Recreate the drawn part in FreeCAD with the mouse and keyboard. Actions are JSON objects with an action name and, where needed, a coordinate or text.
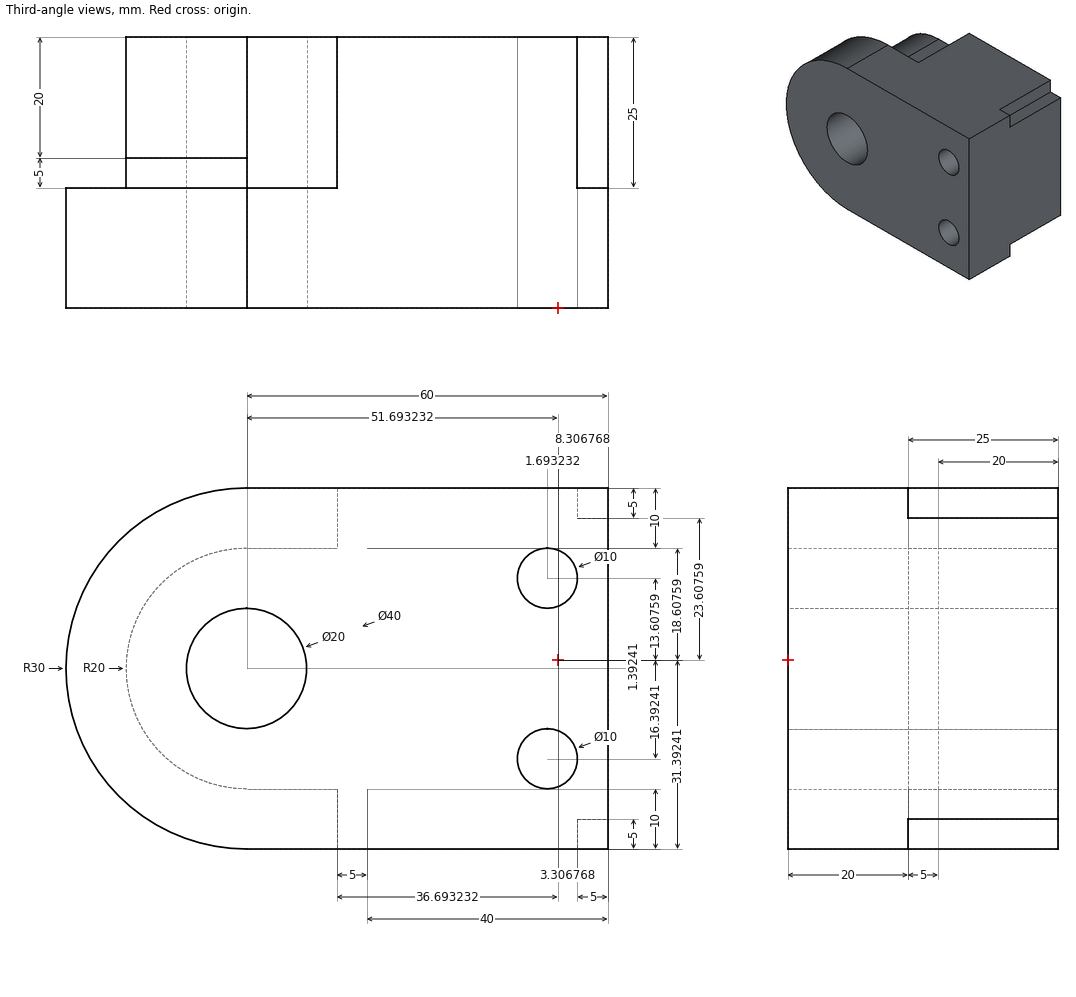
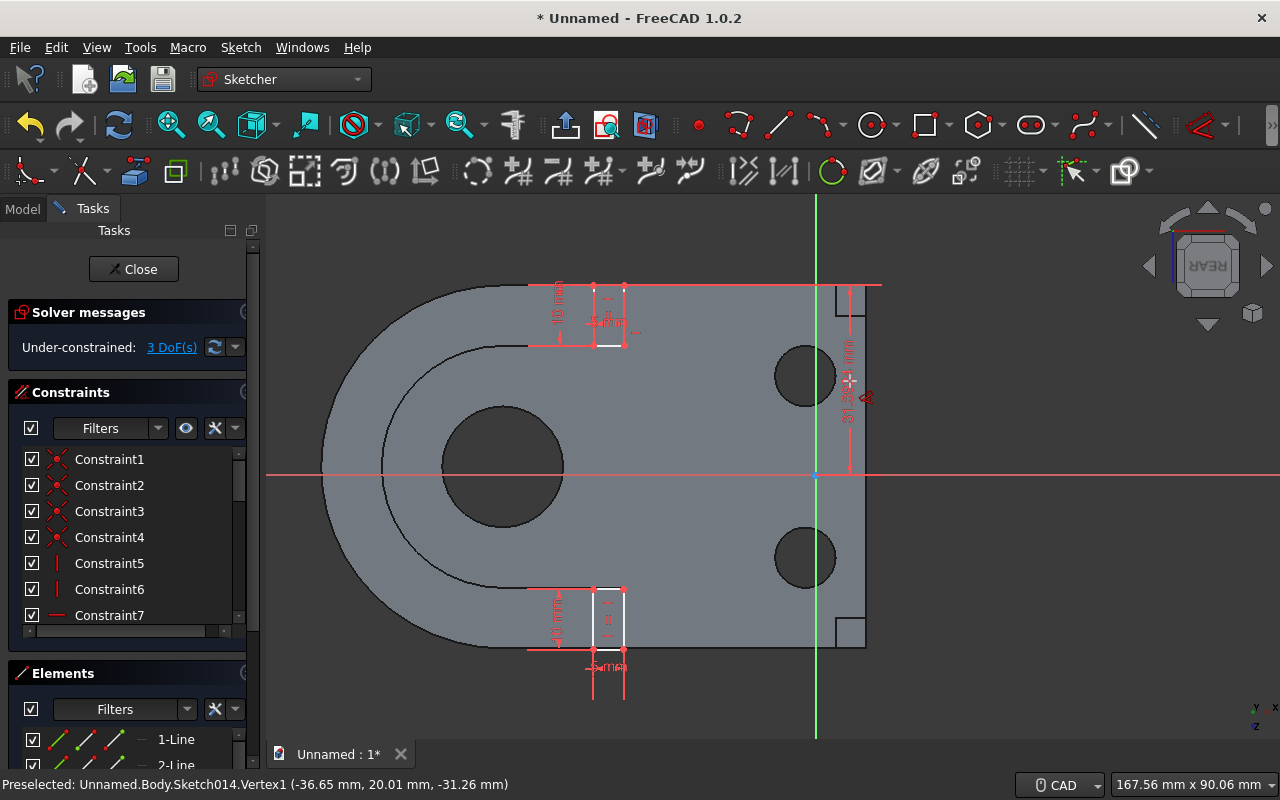
{"action": "left_click", "coordinate": [593, 589]}
{"action": "left_click", "coordinate": [850, 532]}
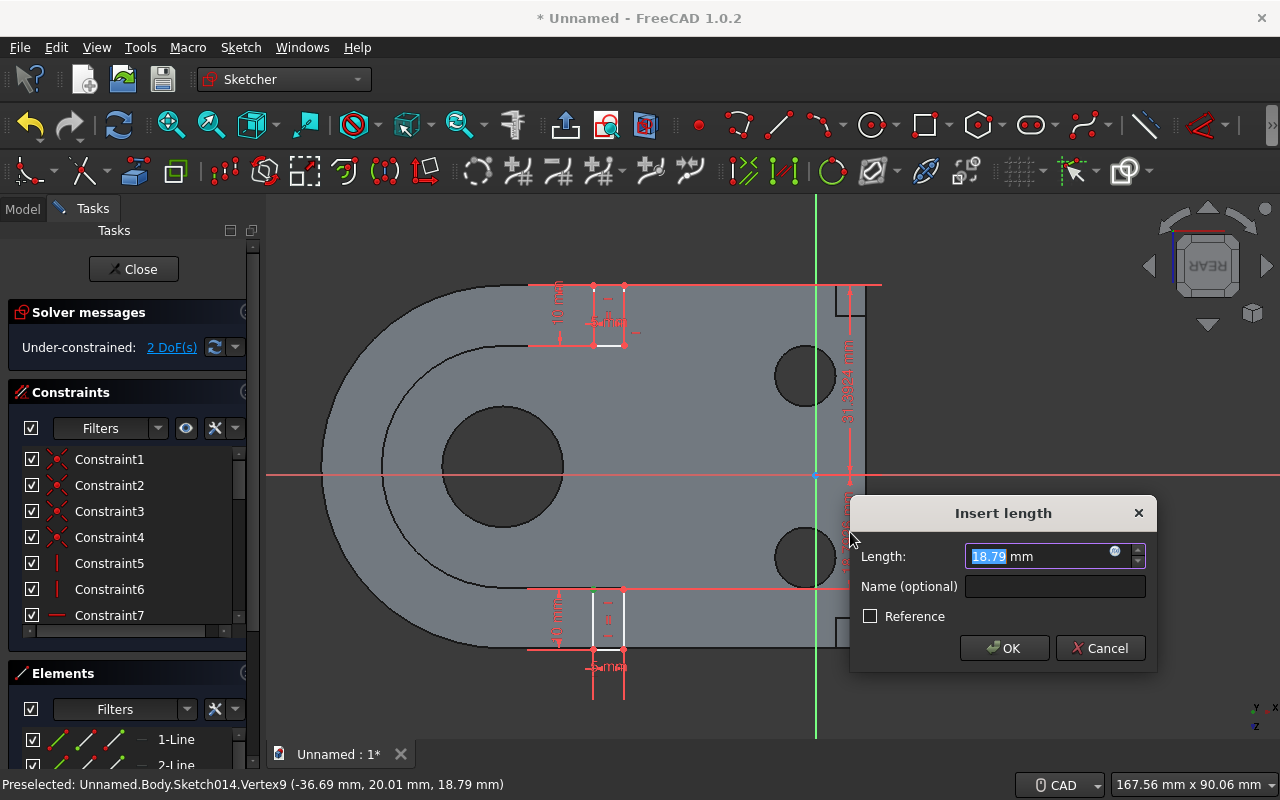
{"action": "type", "text": "18.60759"}
{"action": "key", "text": "Return"}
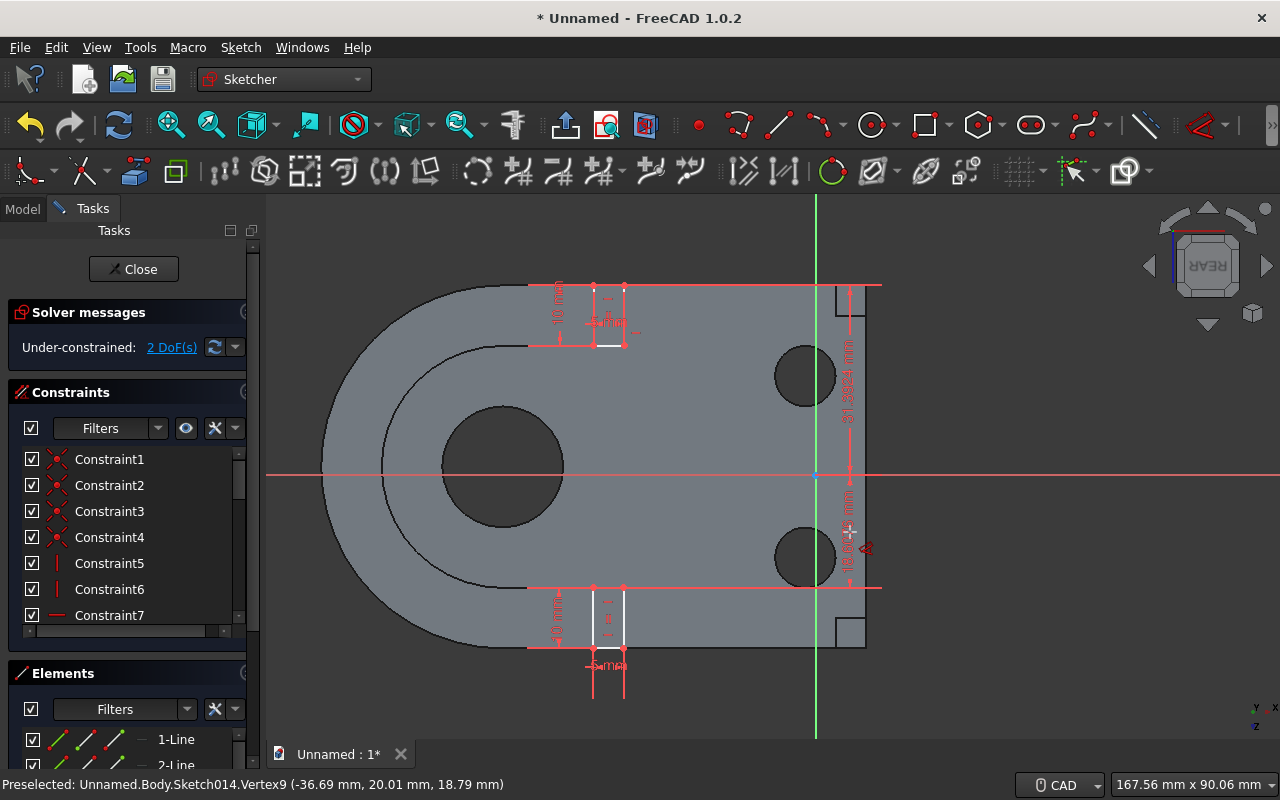
{"action": "left_click", "coordinate": [594, 285]}
{"action": "left_click", "coordinate": [705, 251]}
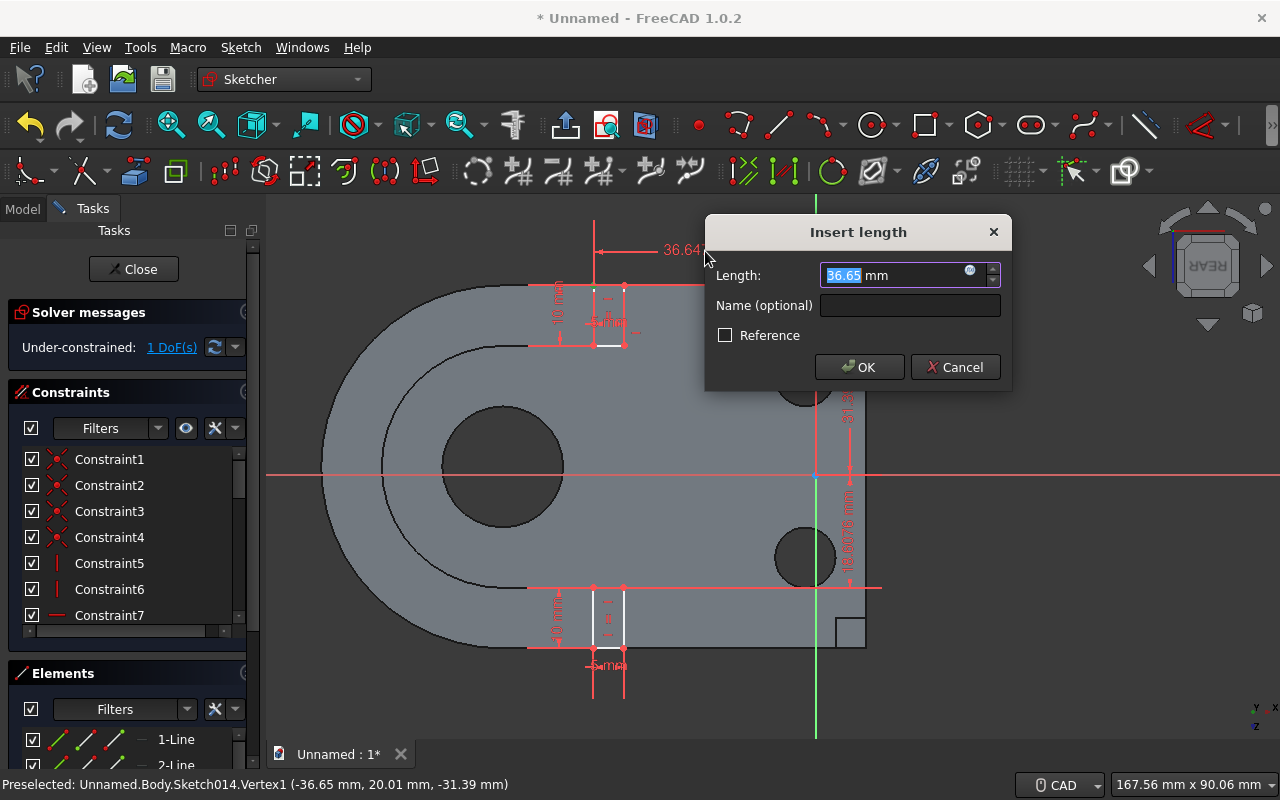
{"action": "type", "text": "36.693232"}
{"action": "key", "text": "Return"}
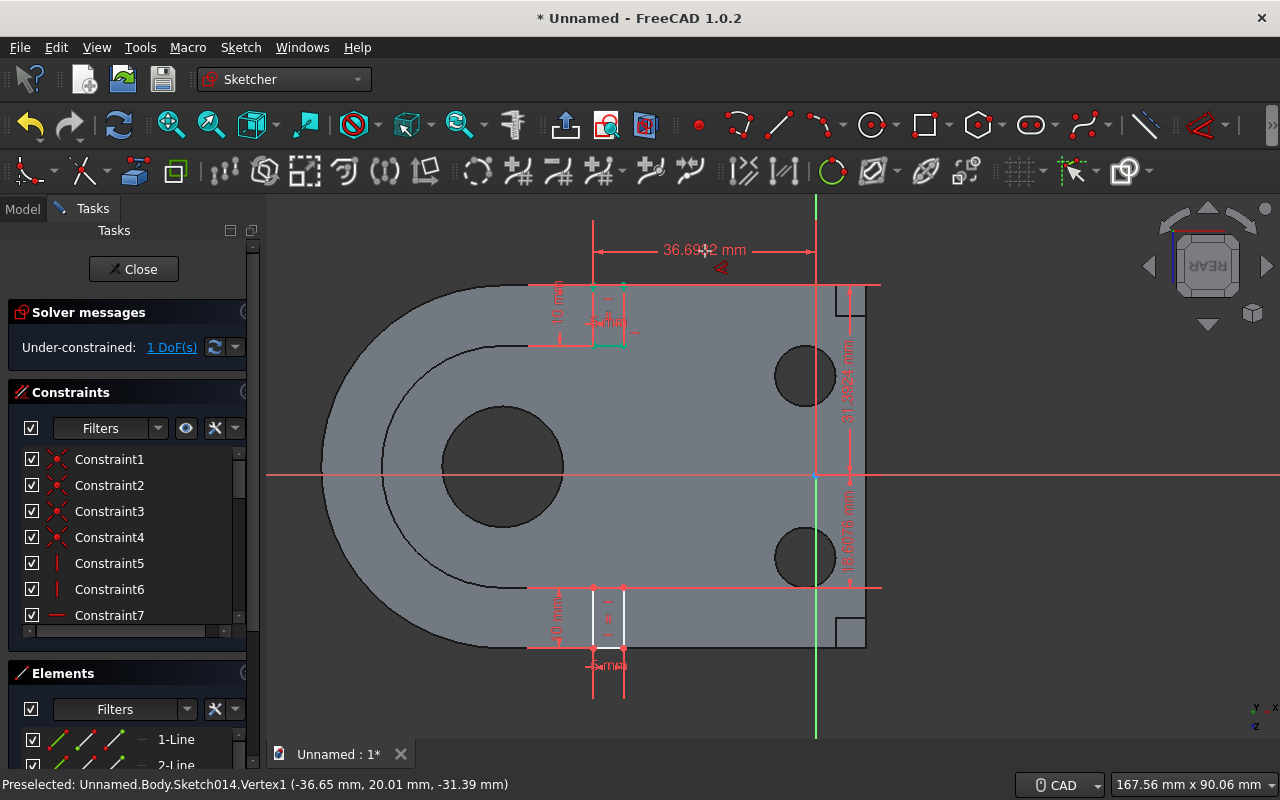
{"action": "left_click", "coordinate": [593, 588]}
{"action": "left_click", "coordinate": [705, 622]}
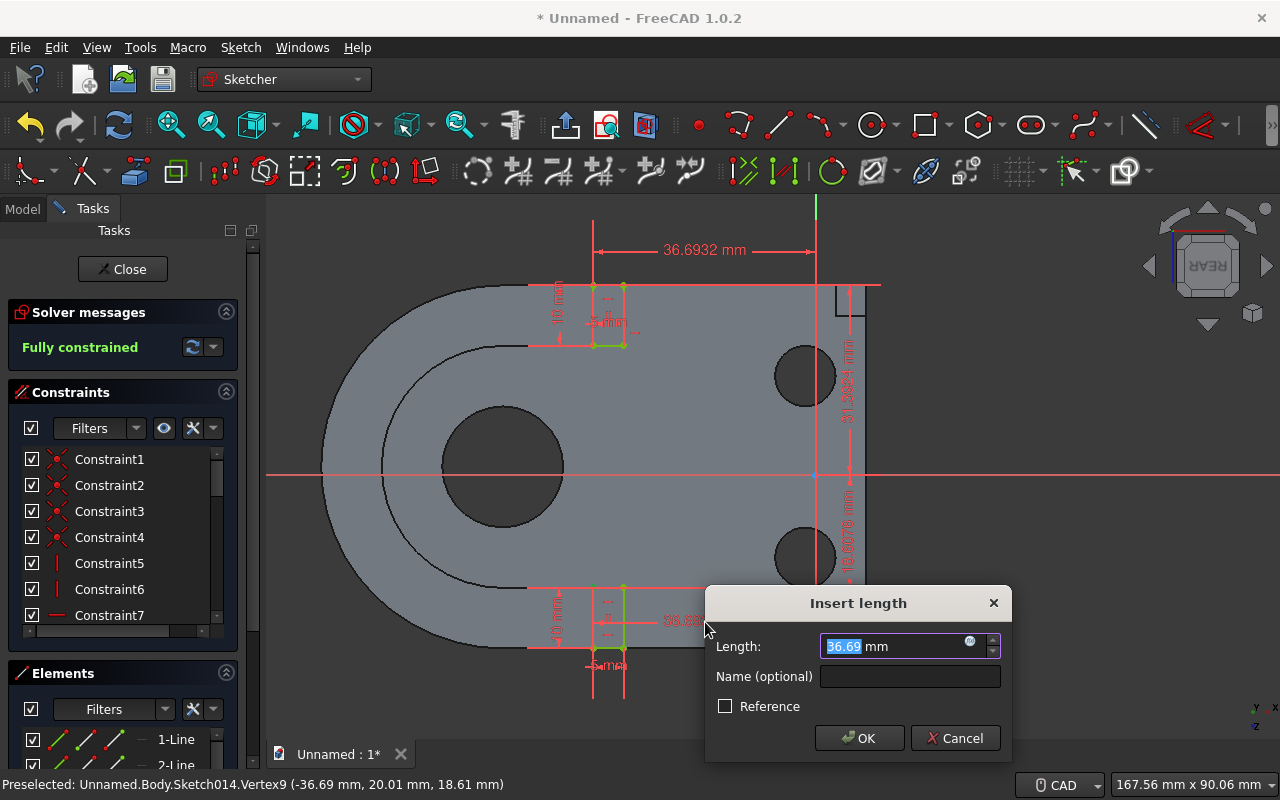
{"action": "type", "text": "36.693232"}
{"action": "key", "text": "Return"}
{"action": "key", "text": "Escape"}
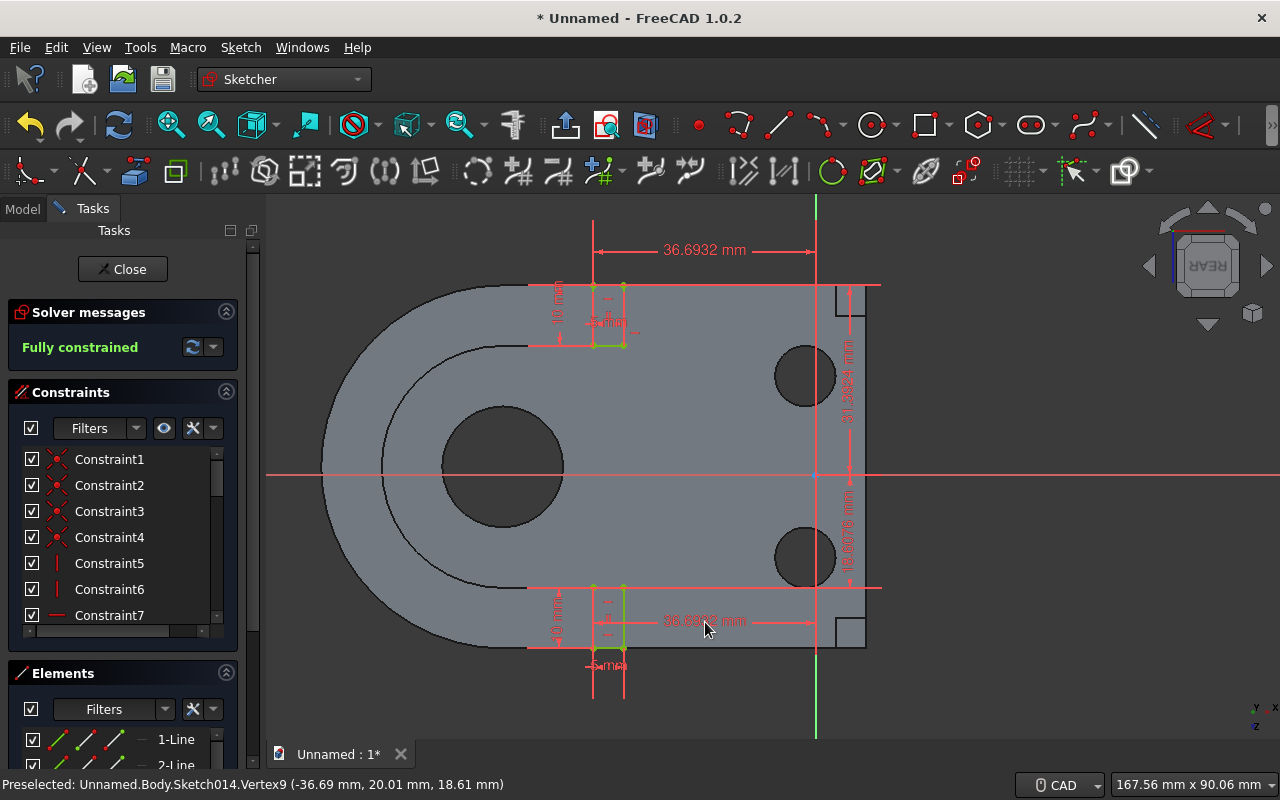
{"action": "left_click", "coordinate": [123, 269]}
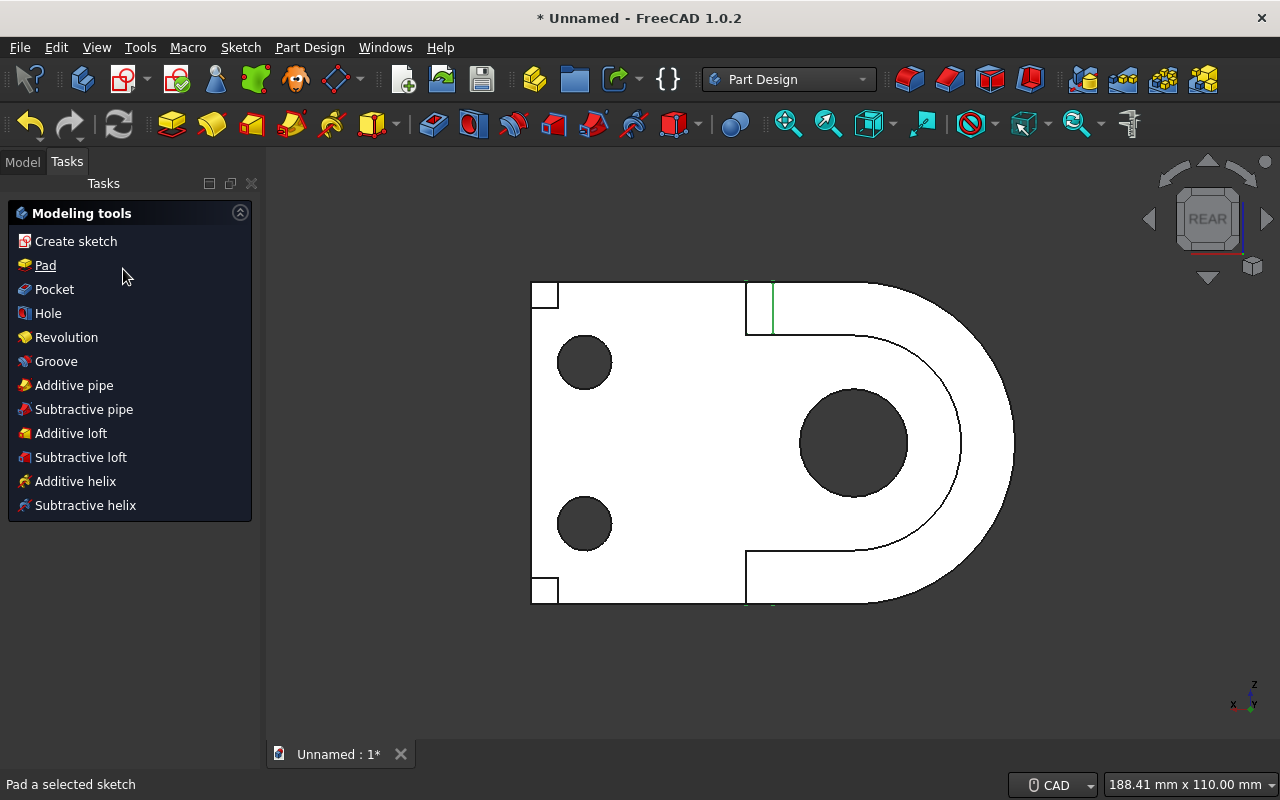
{"action": "left_click", "coordinate": [172, 124]}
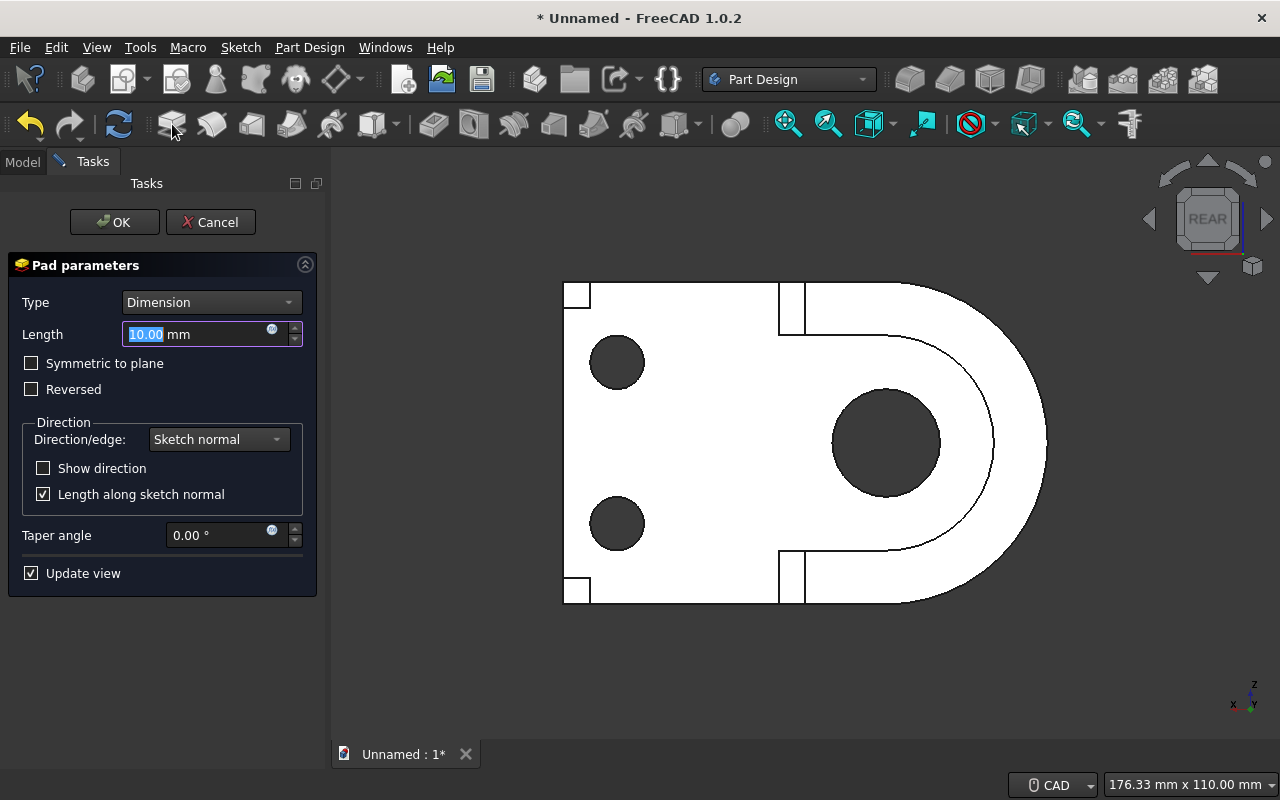
{"action": "type", "text": "25"}
{"action": "key", "text": "Tab"}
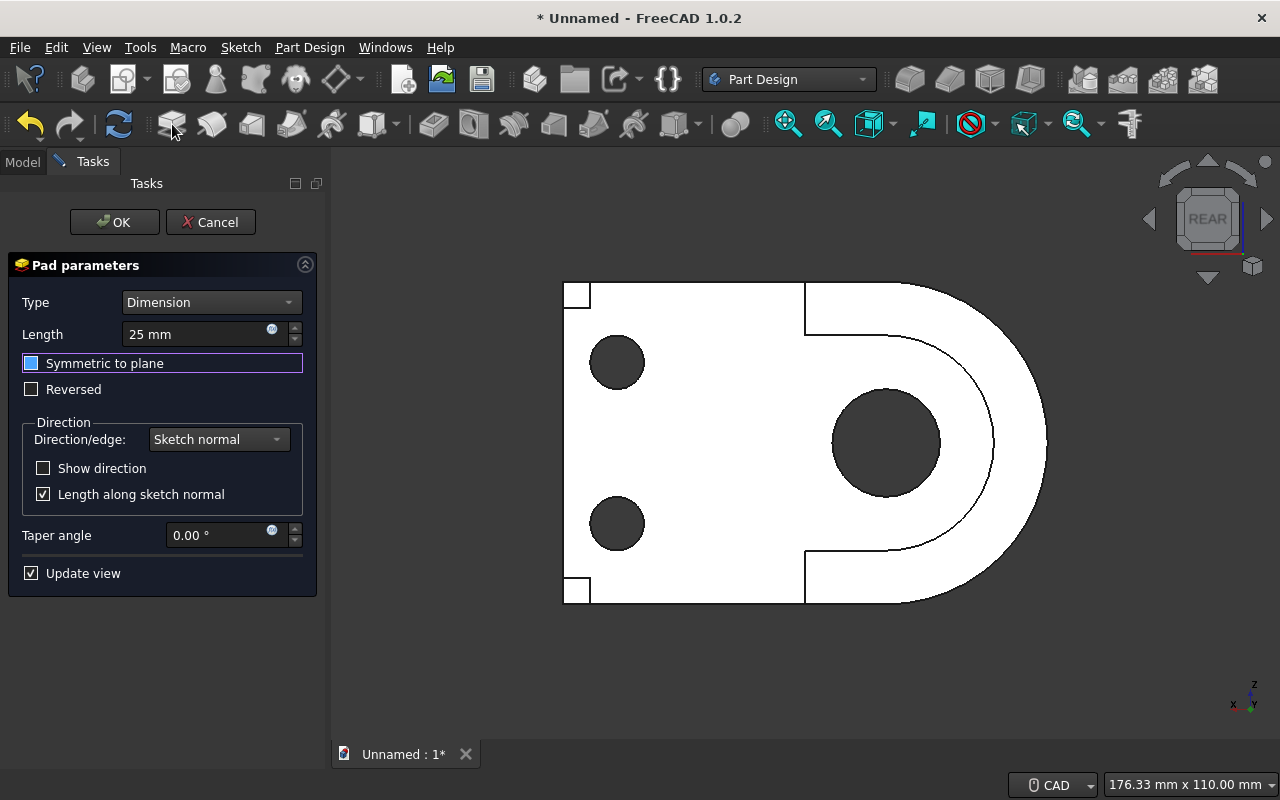
{"action": "left_click", "coordinate": [115, 222]}